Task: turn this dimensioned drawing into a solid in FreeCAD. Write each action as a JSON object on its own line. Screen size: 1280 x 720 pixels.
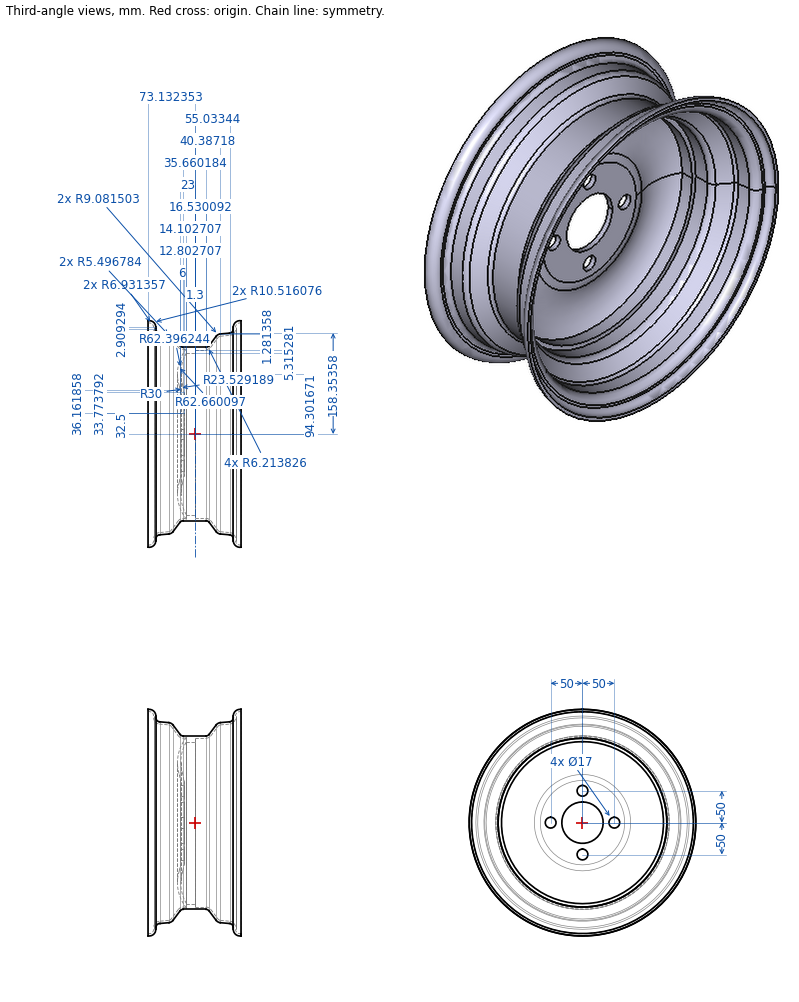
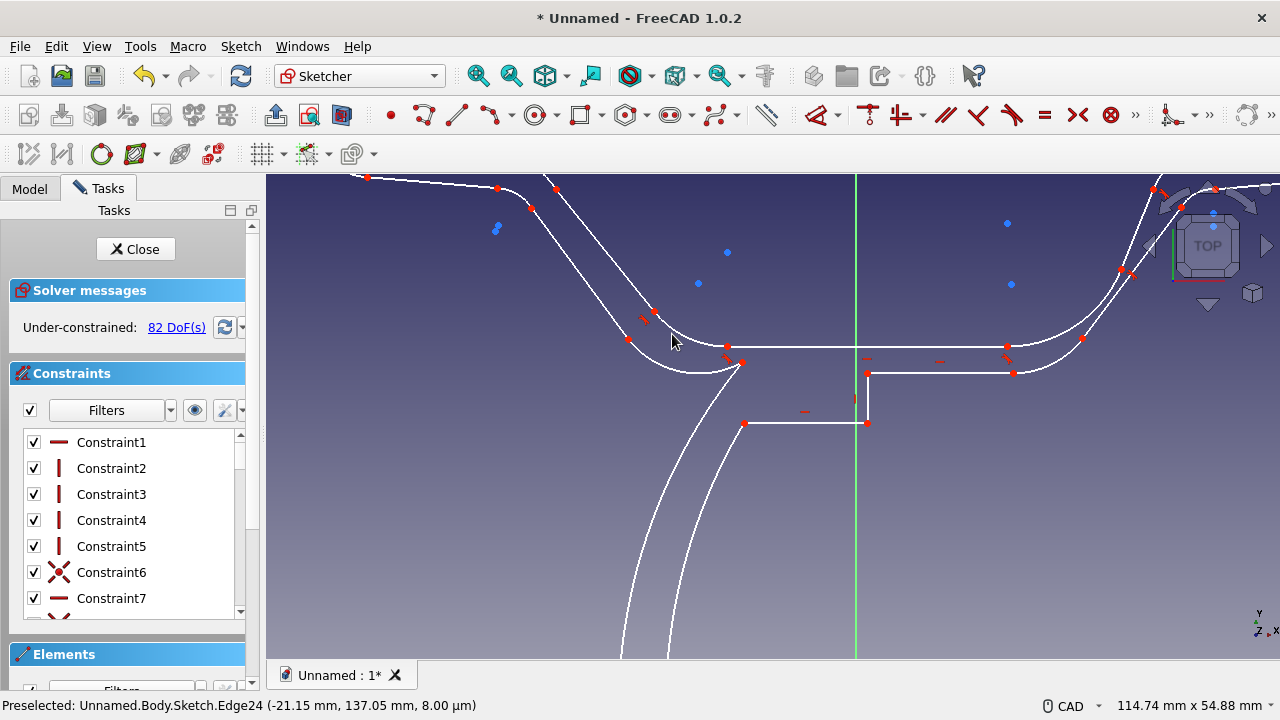
{"action": "left_click", "coordinate": [625, 275]}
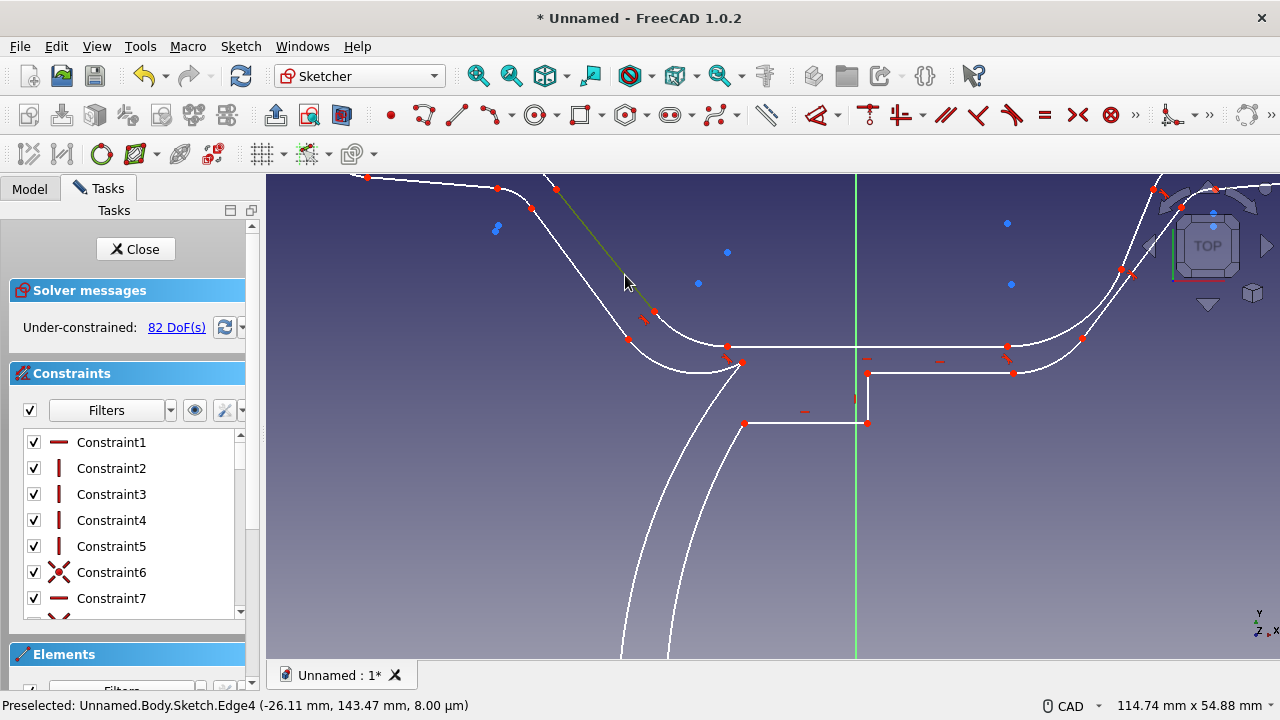
{"action": "scroll", "coordinate": [666, 330], "scroll_direction": "down", "scroll_amount": 8}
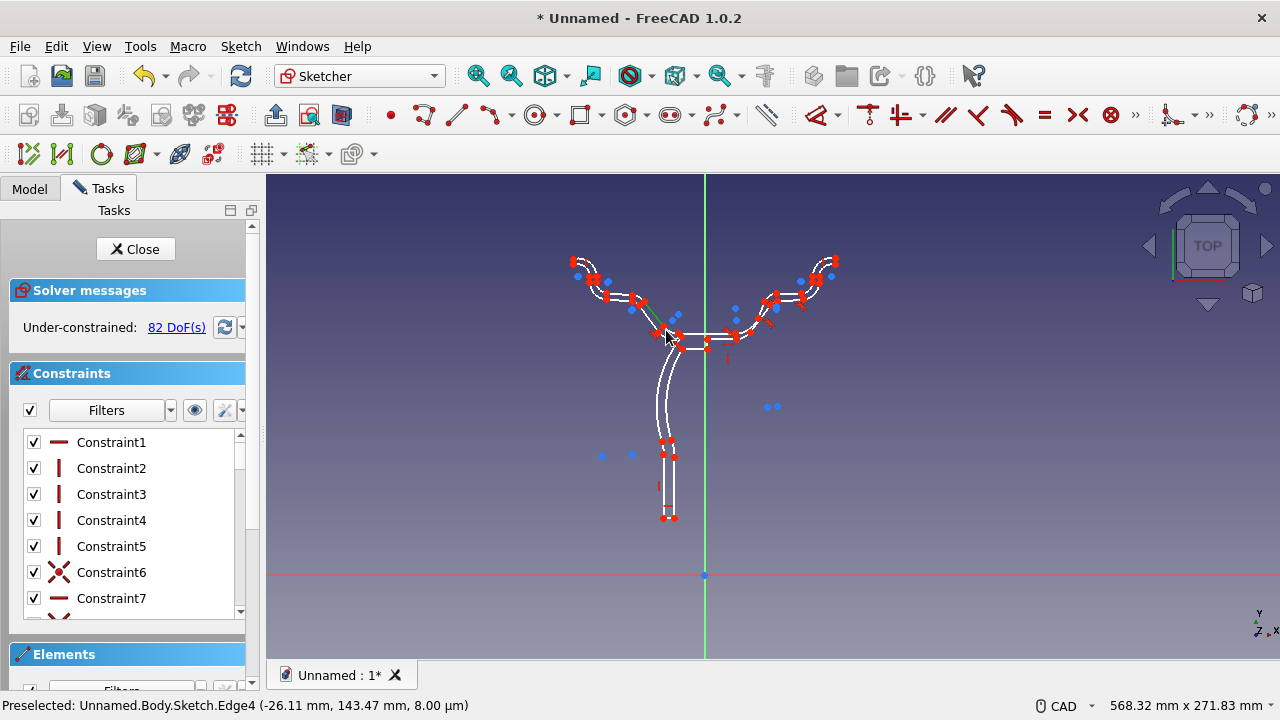
{"action": "scroll", "coordinate": [642, 299], "scroll_direction": "up", "scroll_amount": 7}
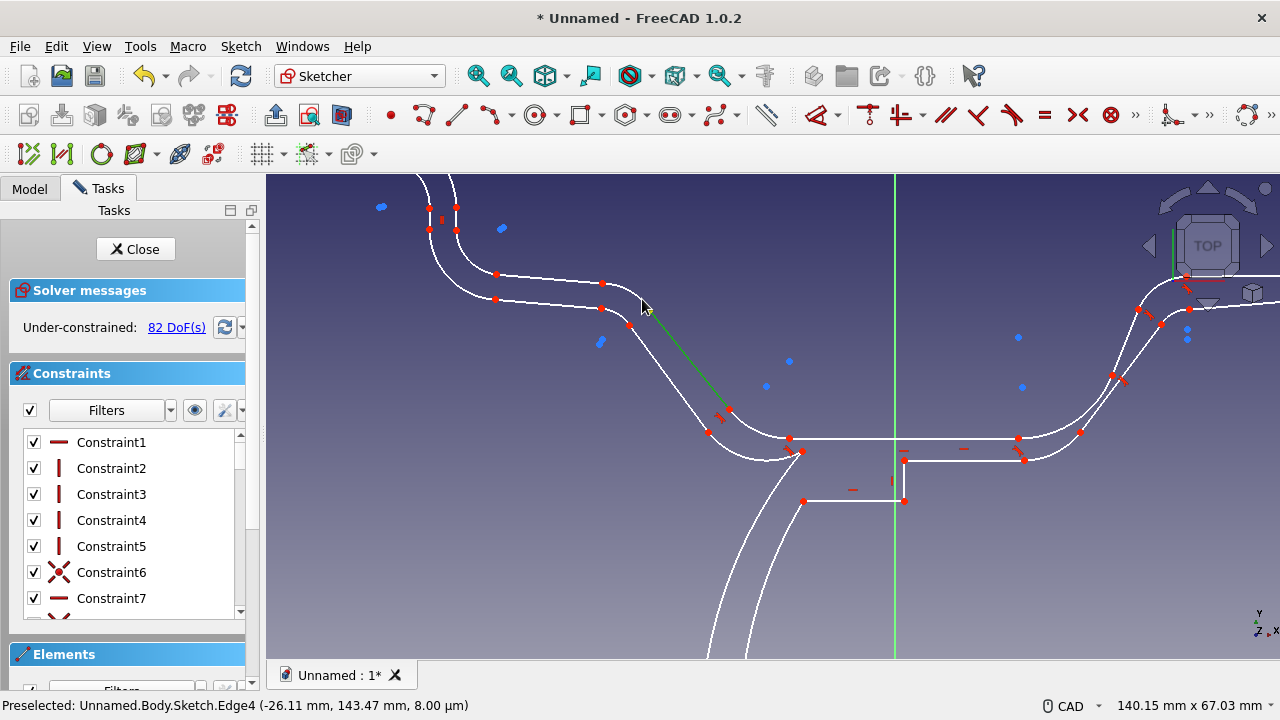
{"action": "left_click", "coordinate": [639, 297]}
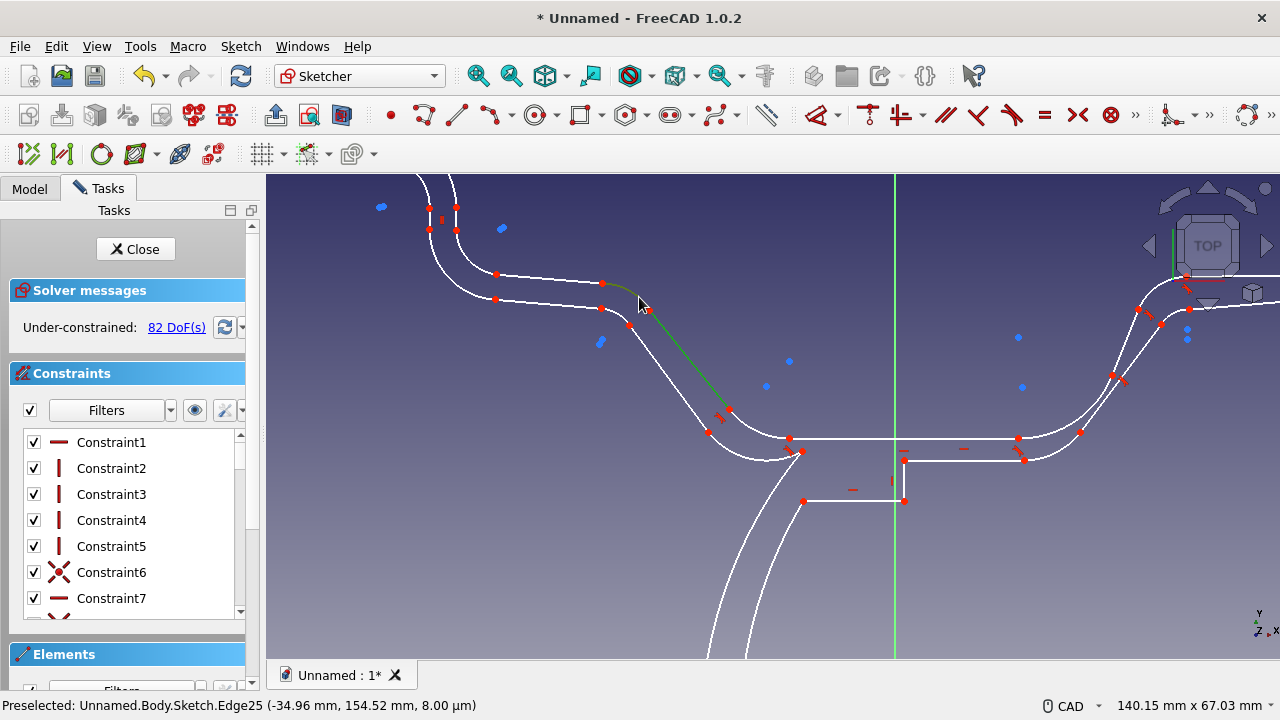
{"action": "key", "text": "t"}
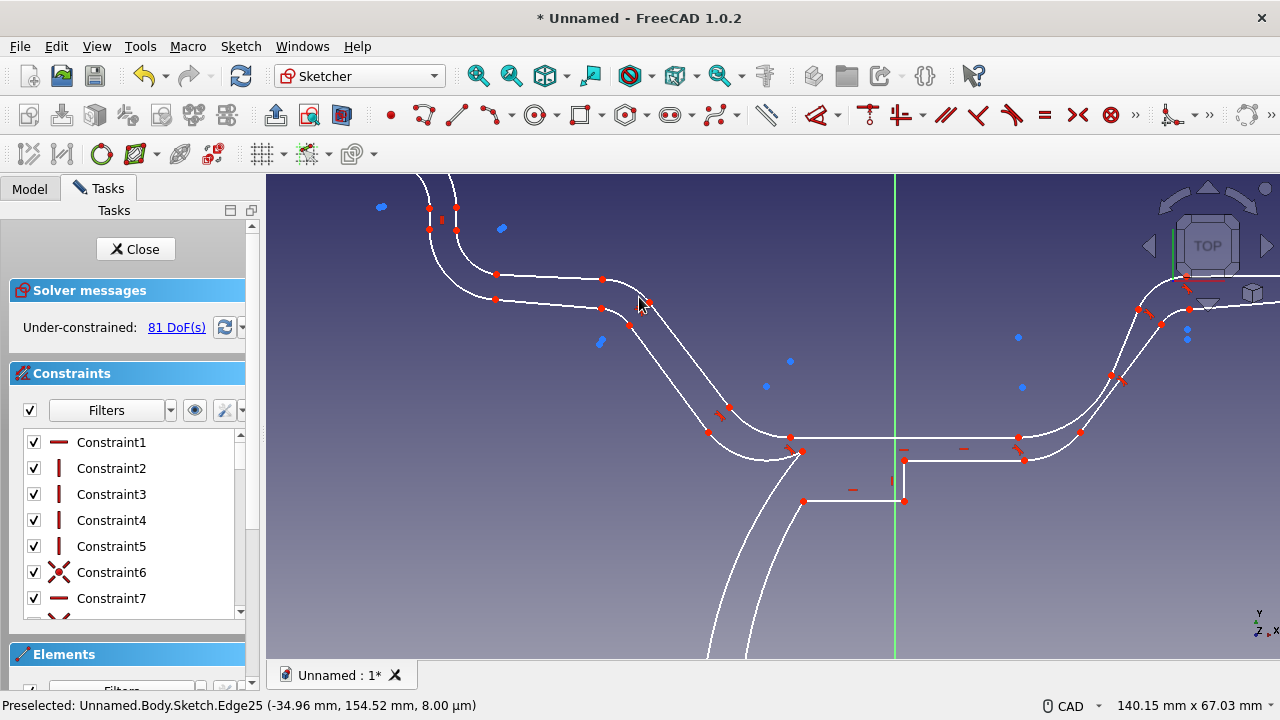
{"action": "left_click", "coordinate": [571, 278]}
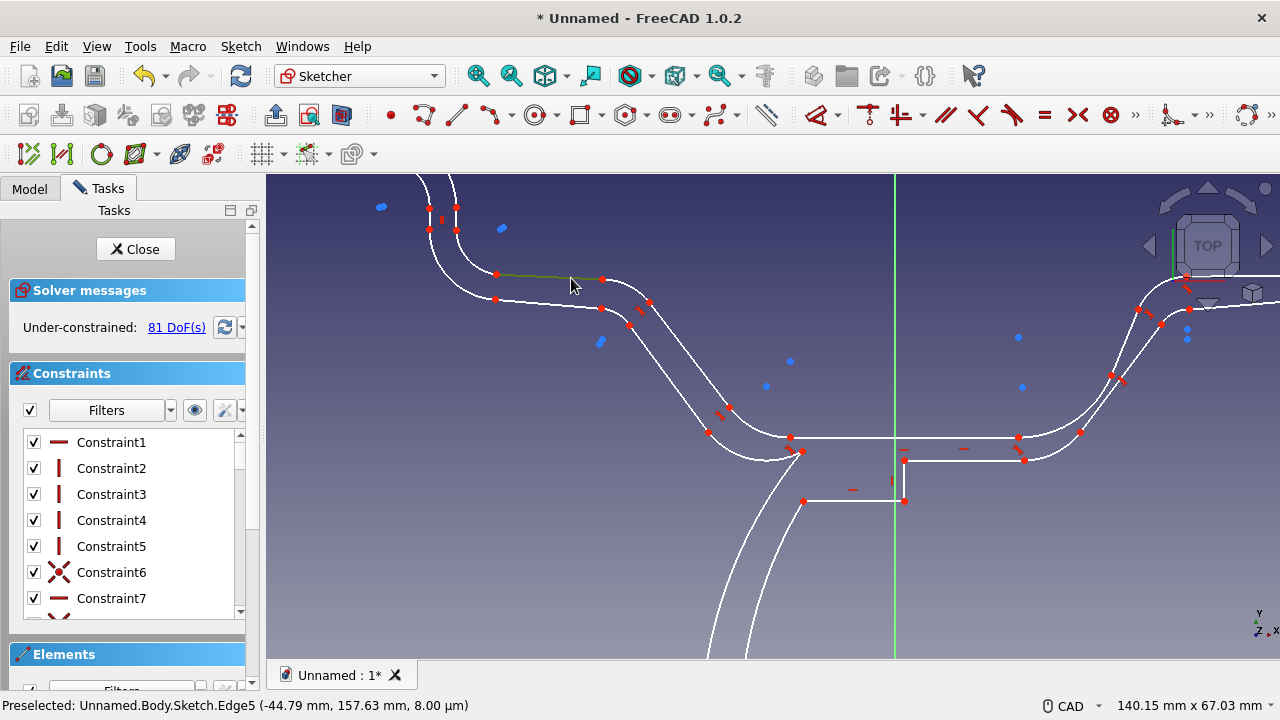
{"action": "left_click", "coordinate": [638, 292]}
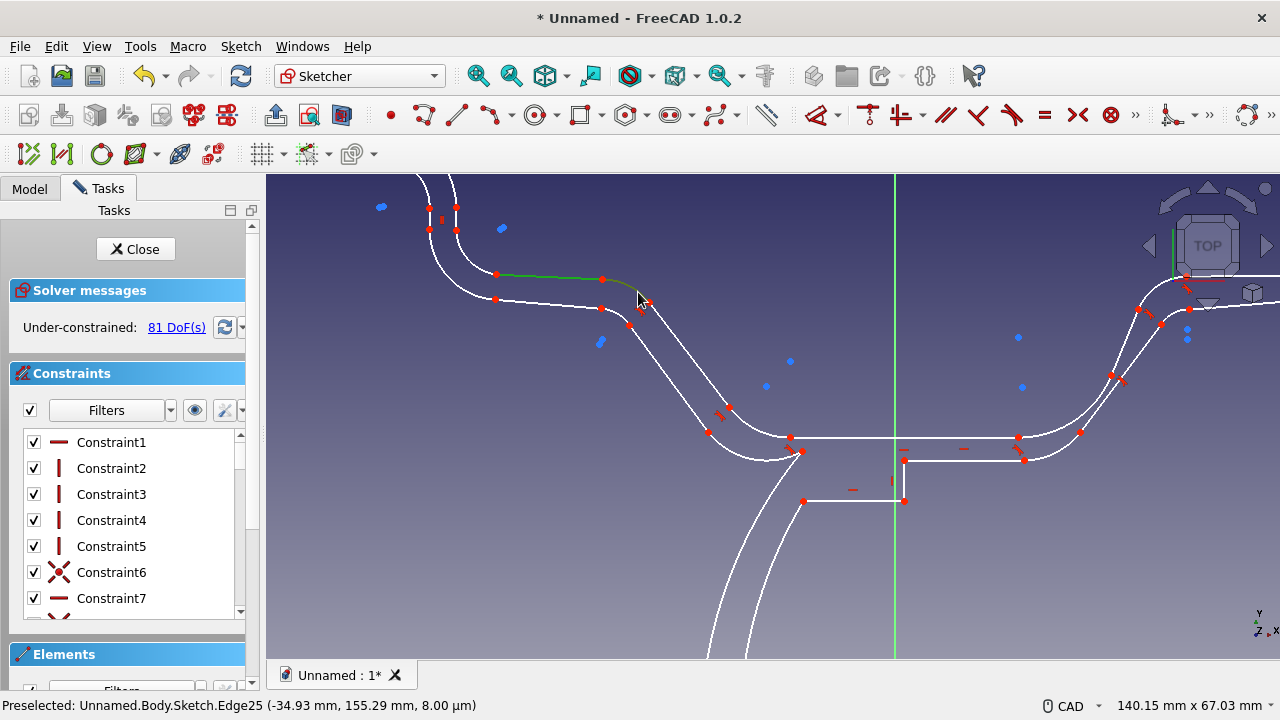
{"action": "key", "text": "t"}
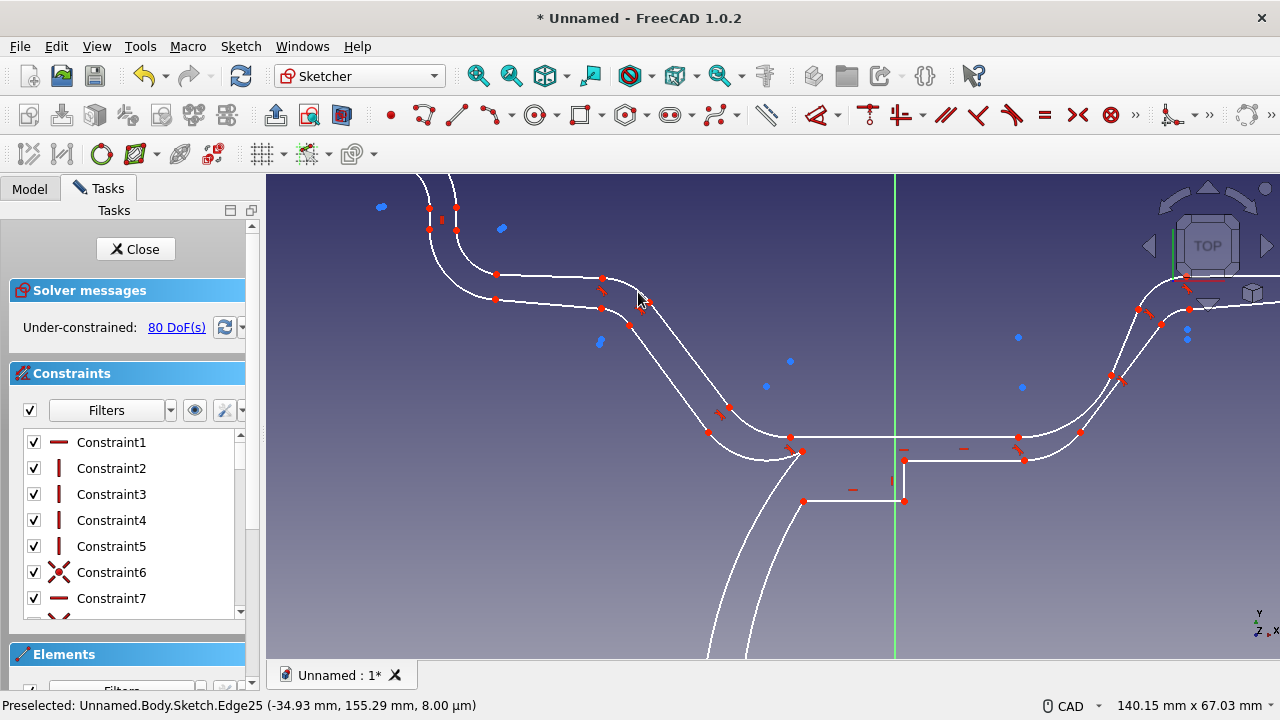
{"action": "left_click", "coordinate": [571, 277]}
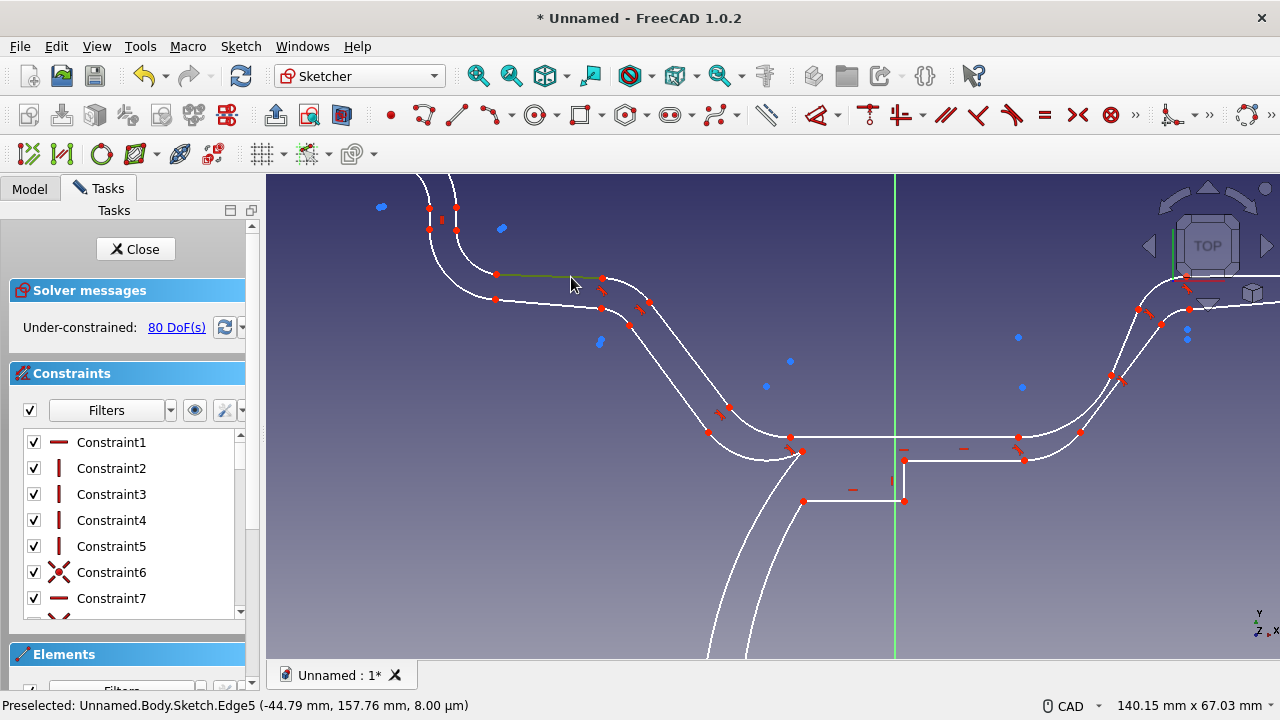
{"action": "left_click", "coordinate": [461, 249]}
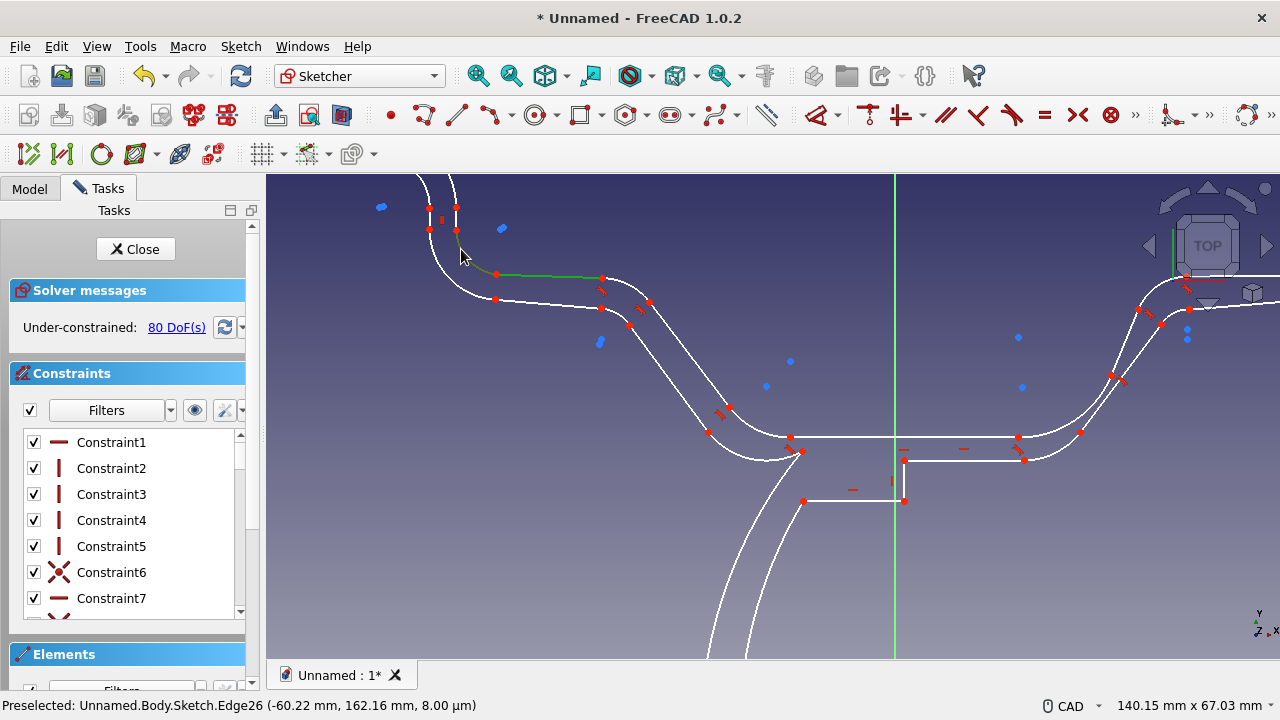
{"action": "key", "text": "t"}